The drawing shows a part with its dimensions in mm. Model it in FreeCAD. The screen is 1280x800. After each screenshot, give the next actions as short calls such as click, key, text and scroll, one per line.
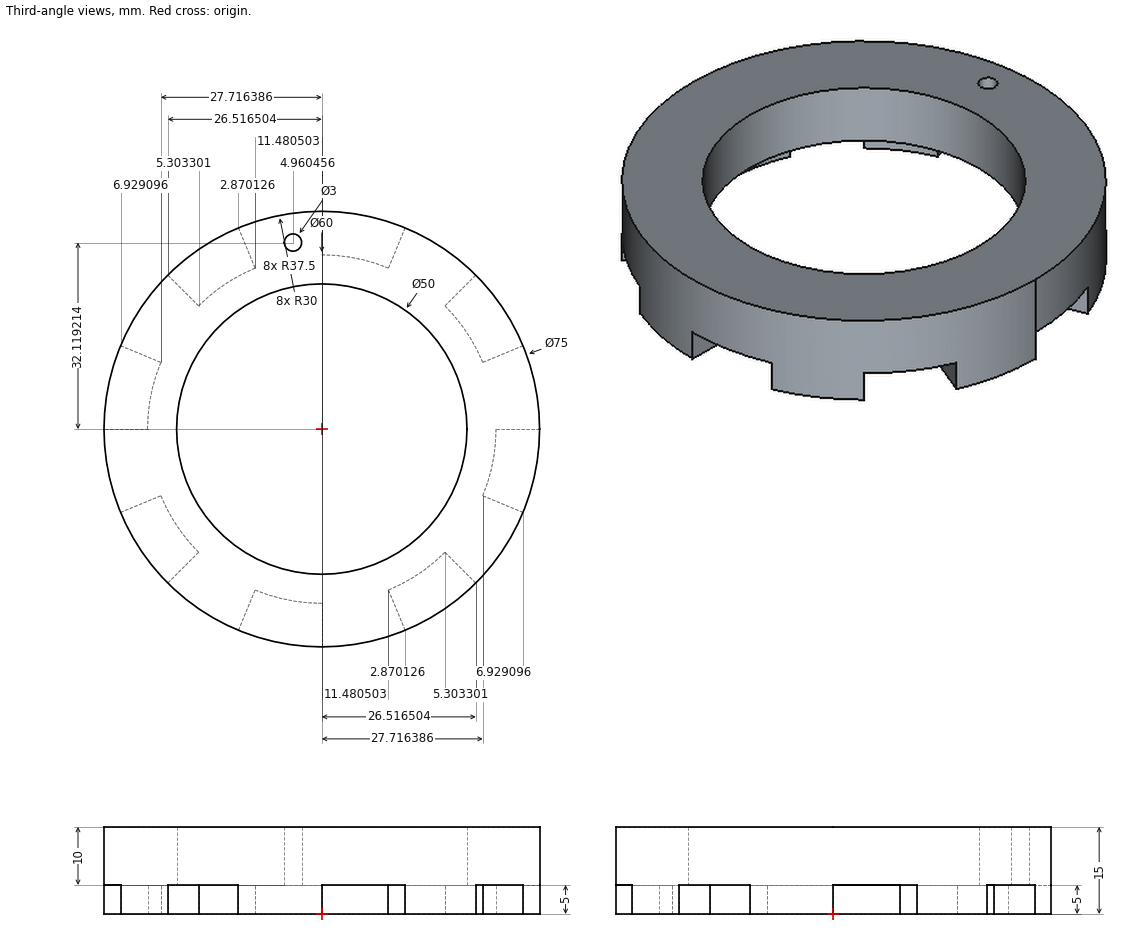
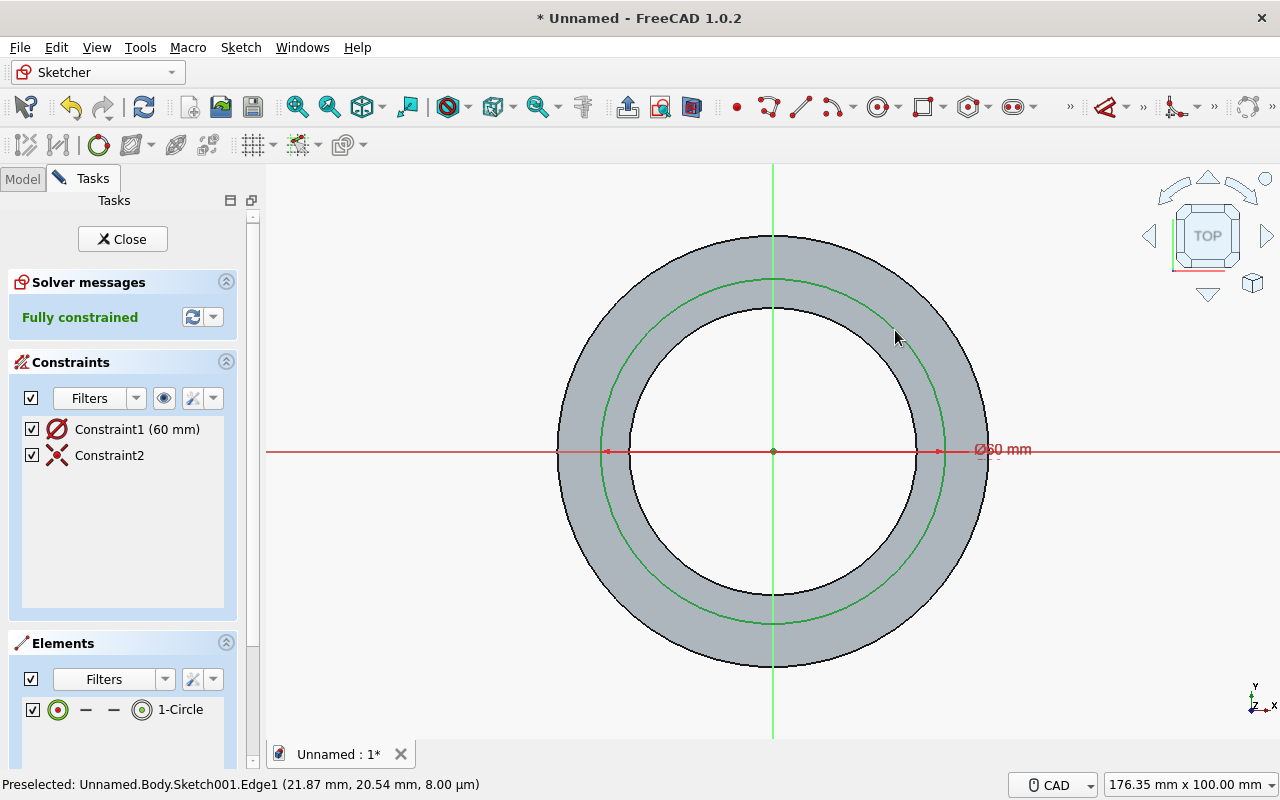
click(123, 239)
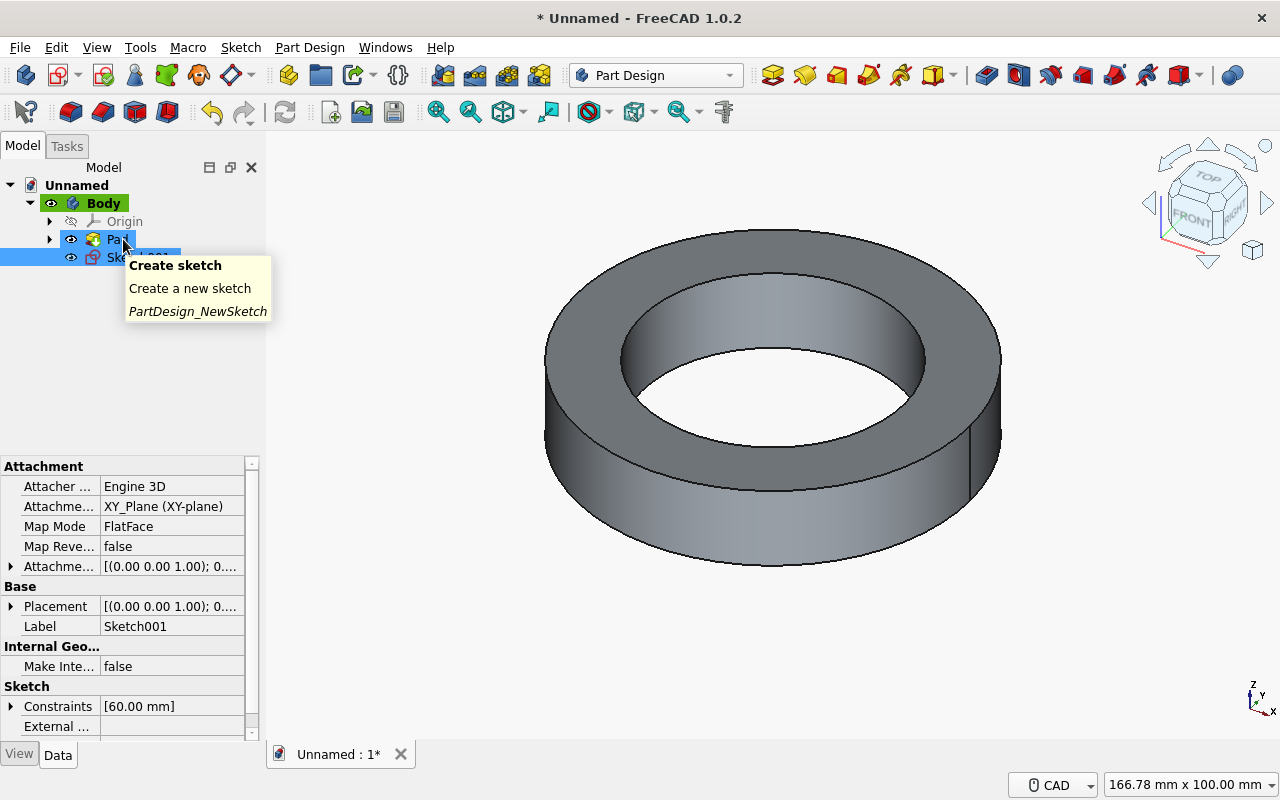
click(988, 76)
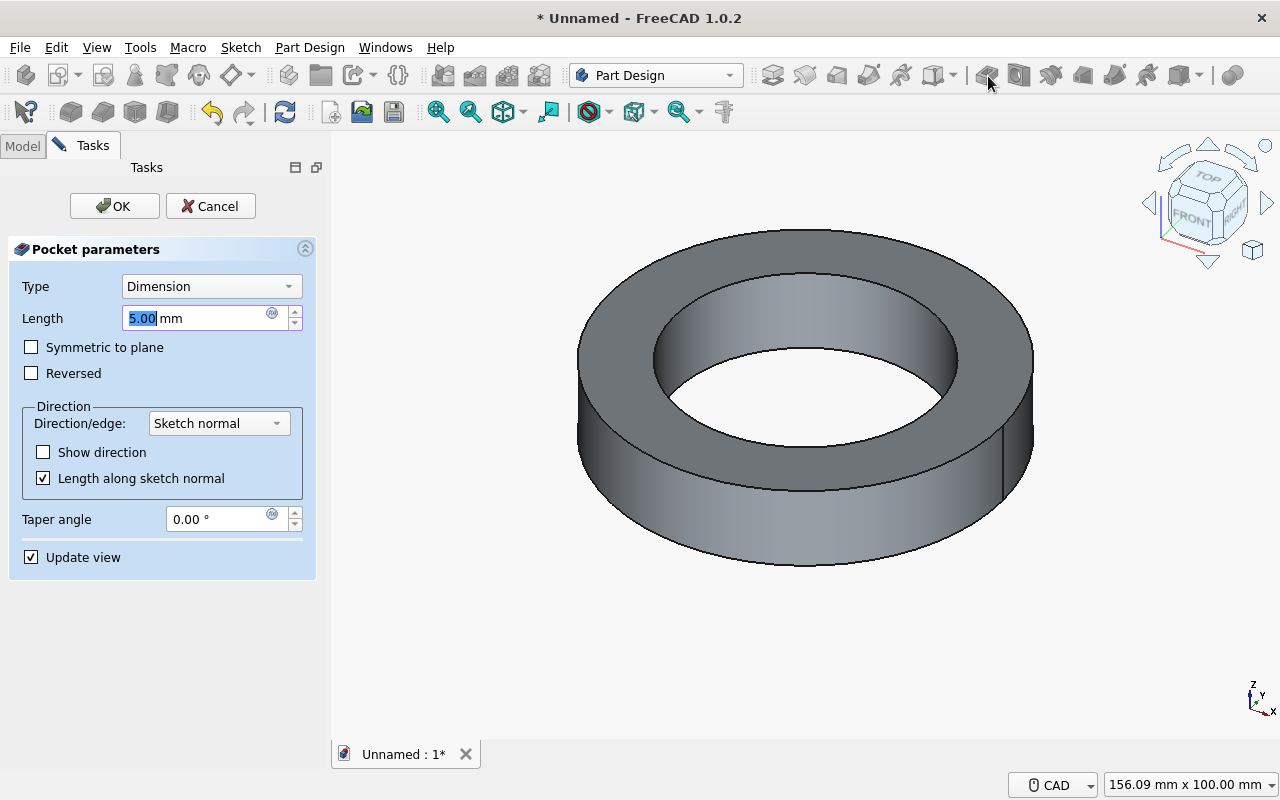
text(5)
key(Tab)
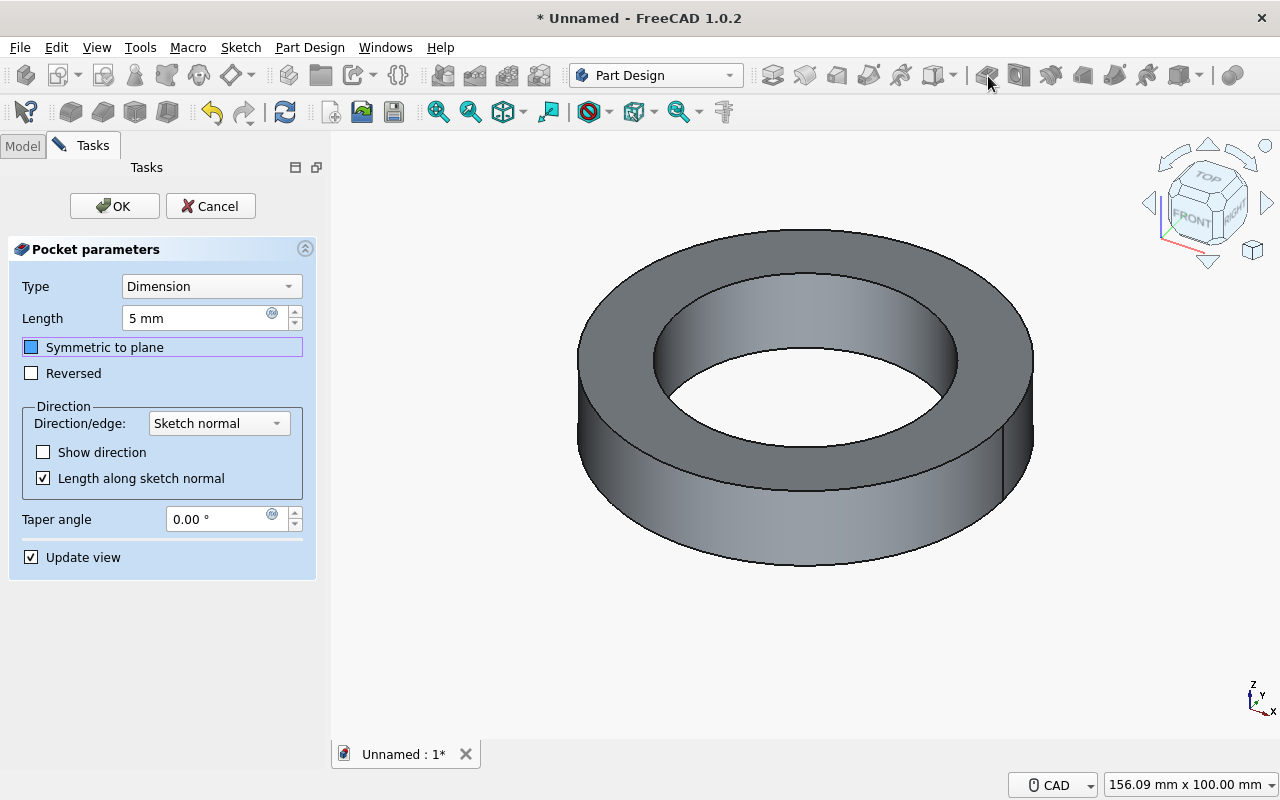
click(30, 373)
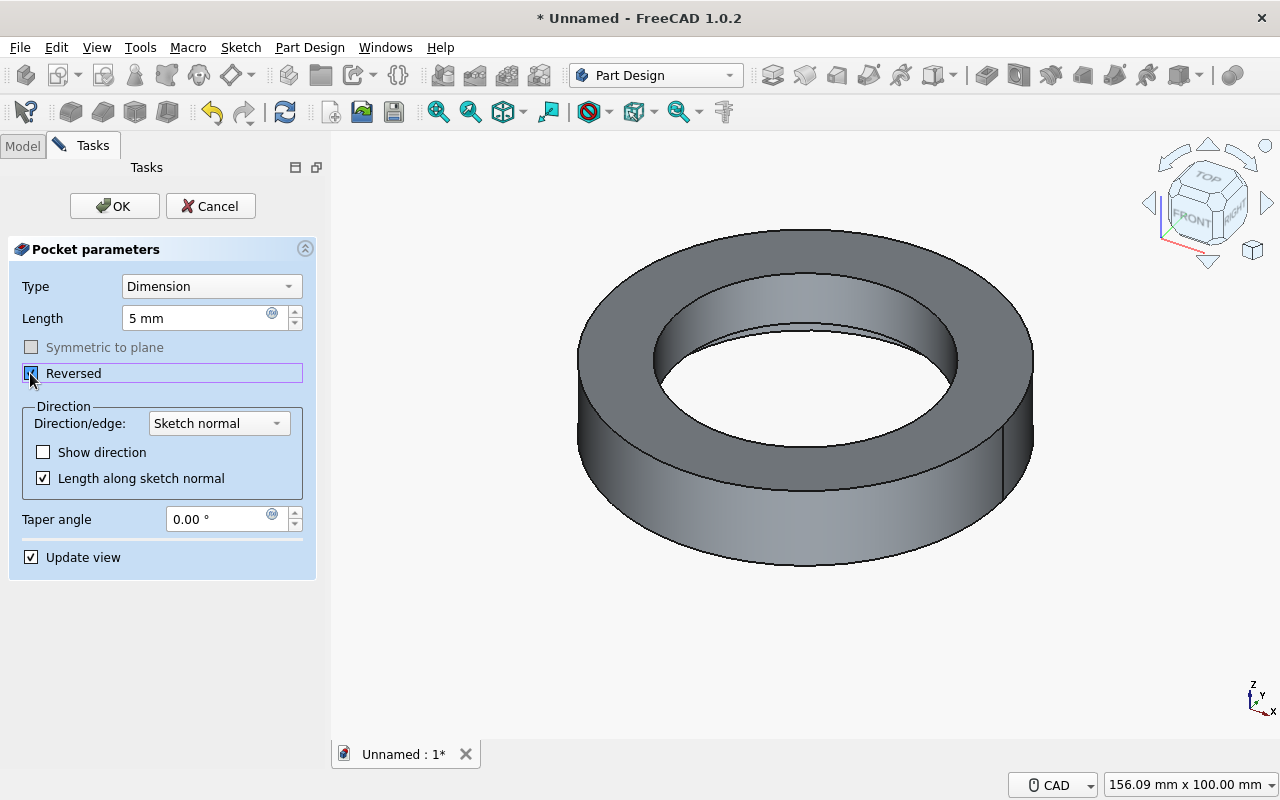
click(115, 206)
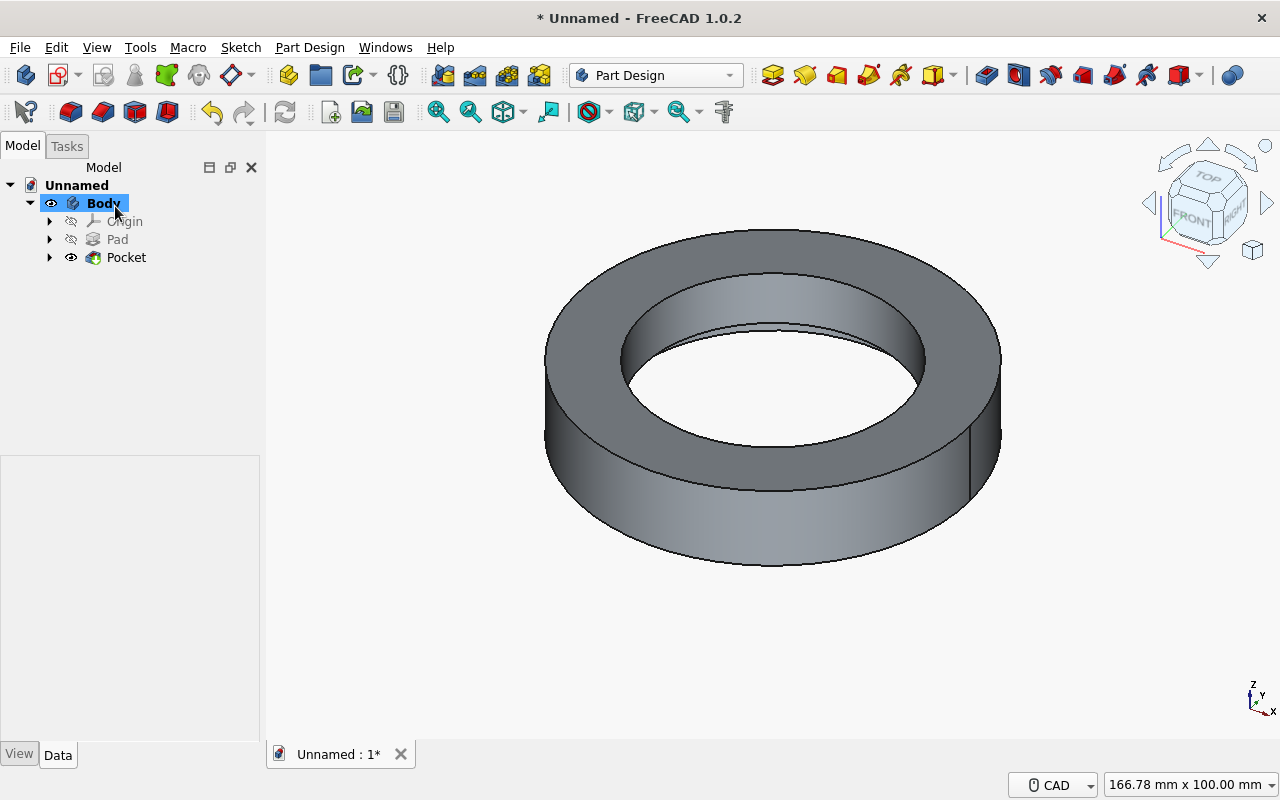
key(5)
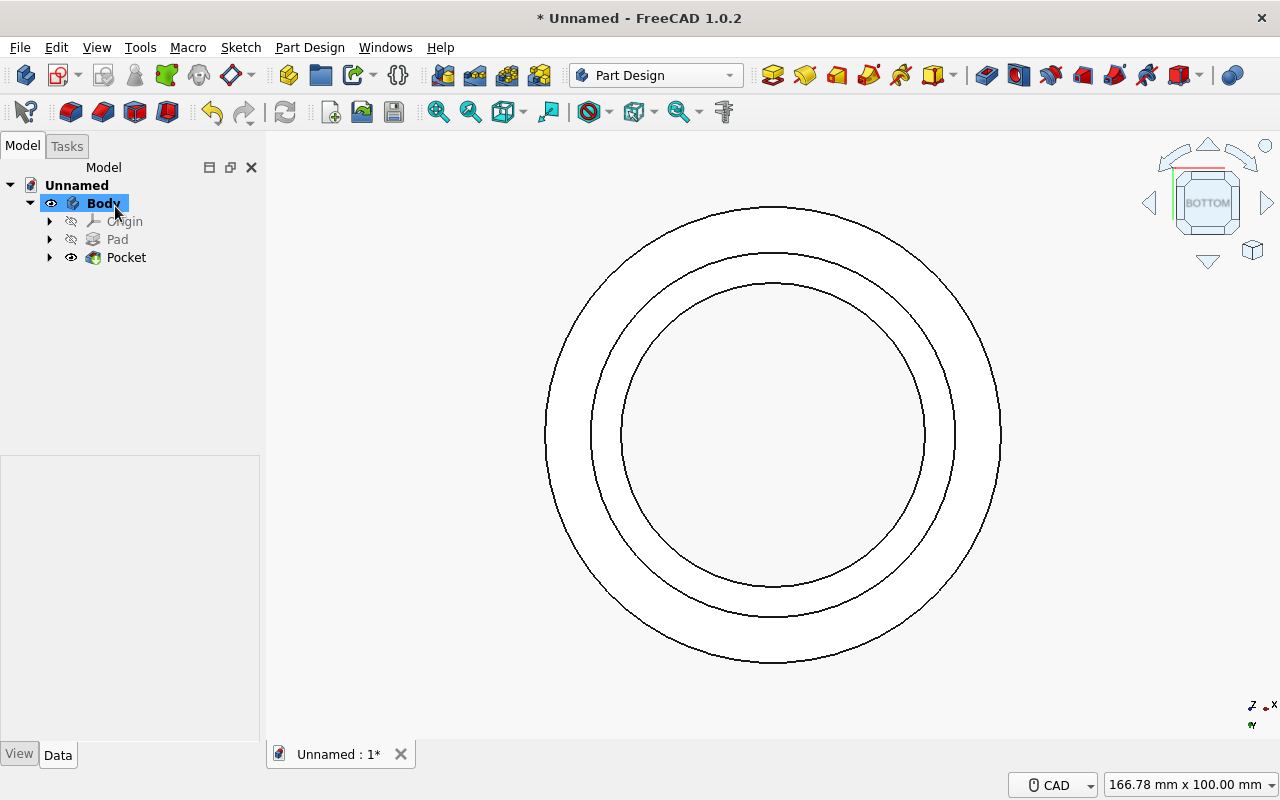
click(968, 369)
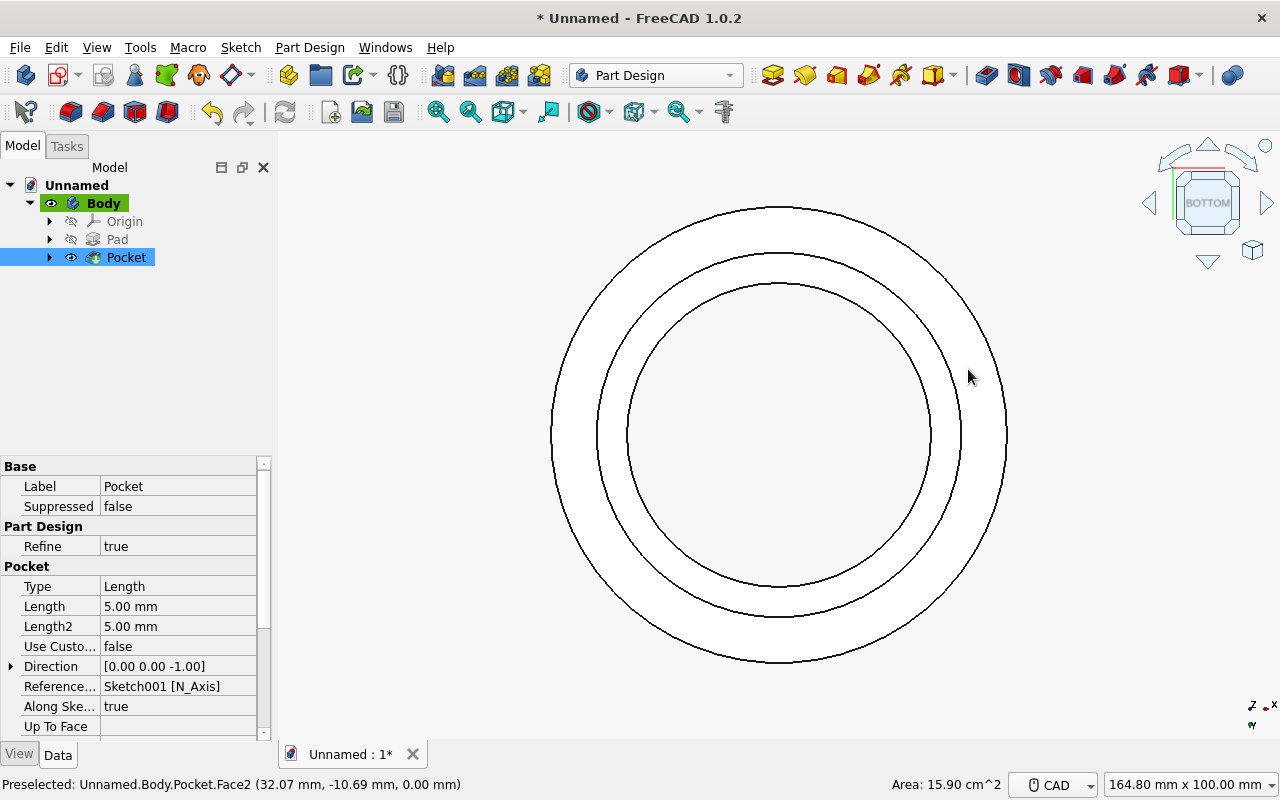
click(58, 76)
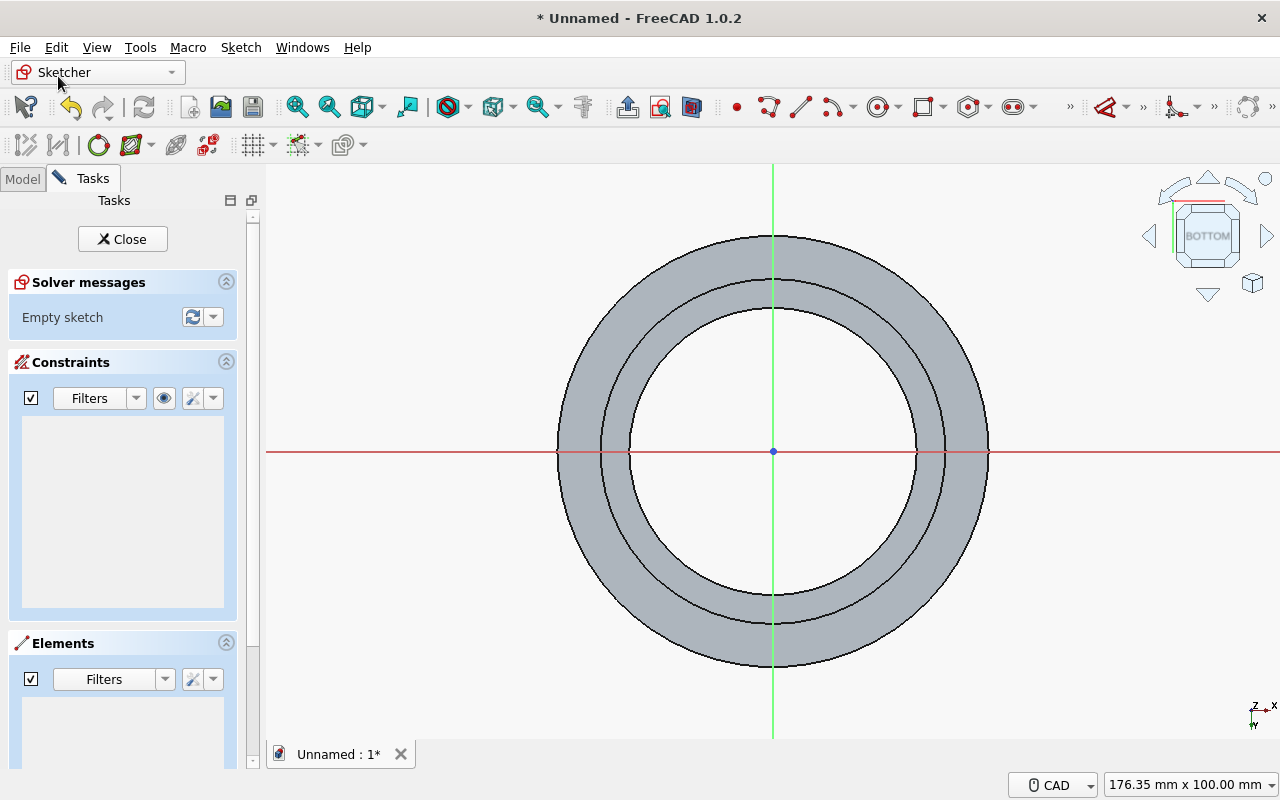
key(g)
key(l)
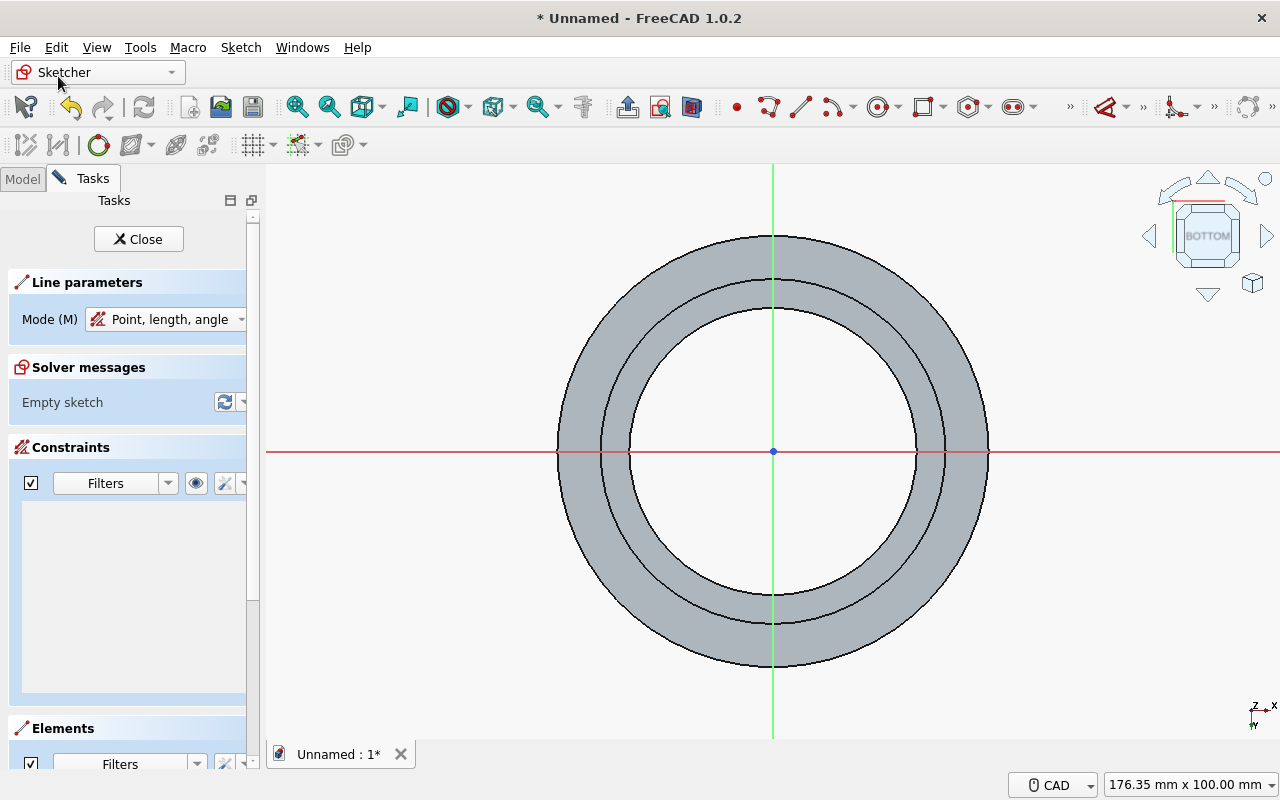
click(773, 667)
click(782, 624)